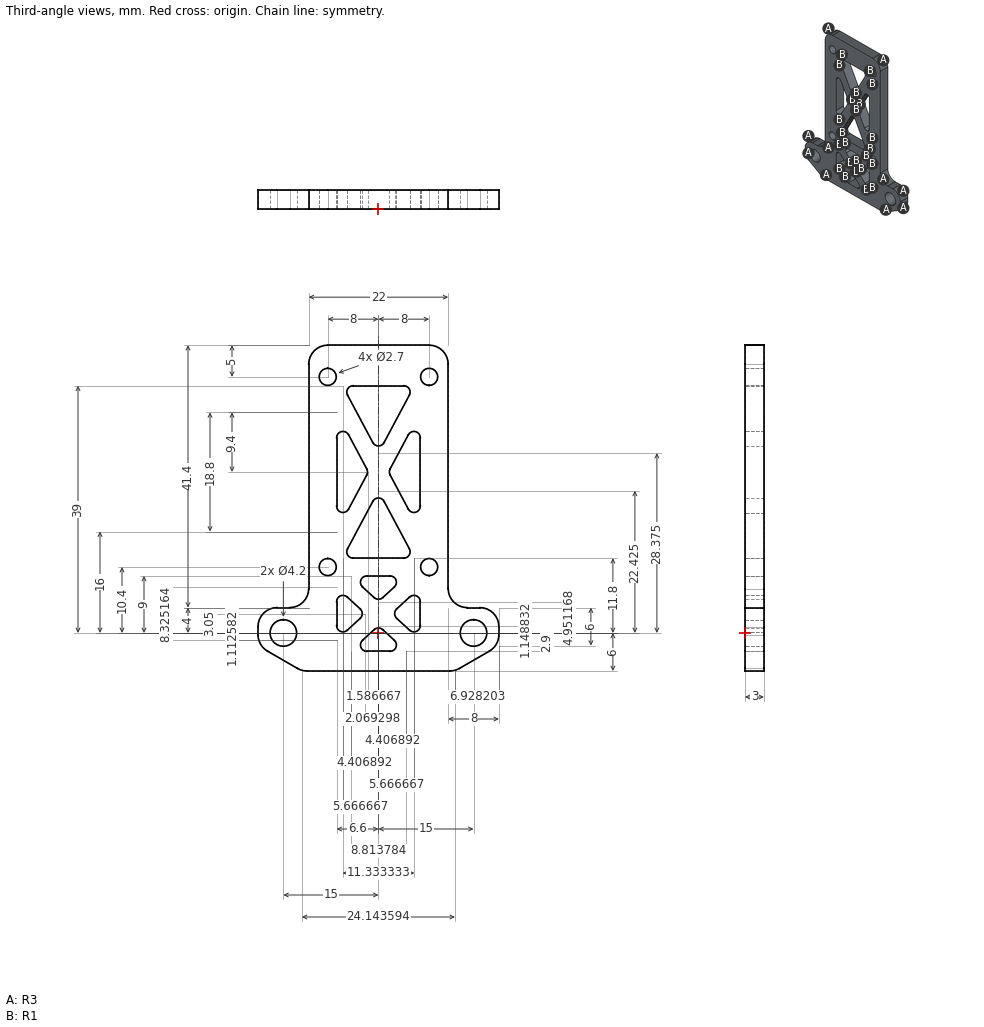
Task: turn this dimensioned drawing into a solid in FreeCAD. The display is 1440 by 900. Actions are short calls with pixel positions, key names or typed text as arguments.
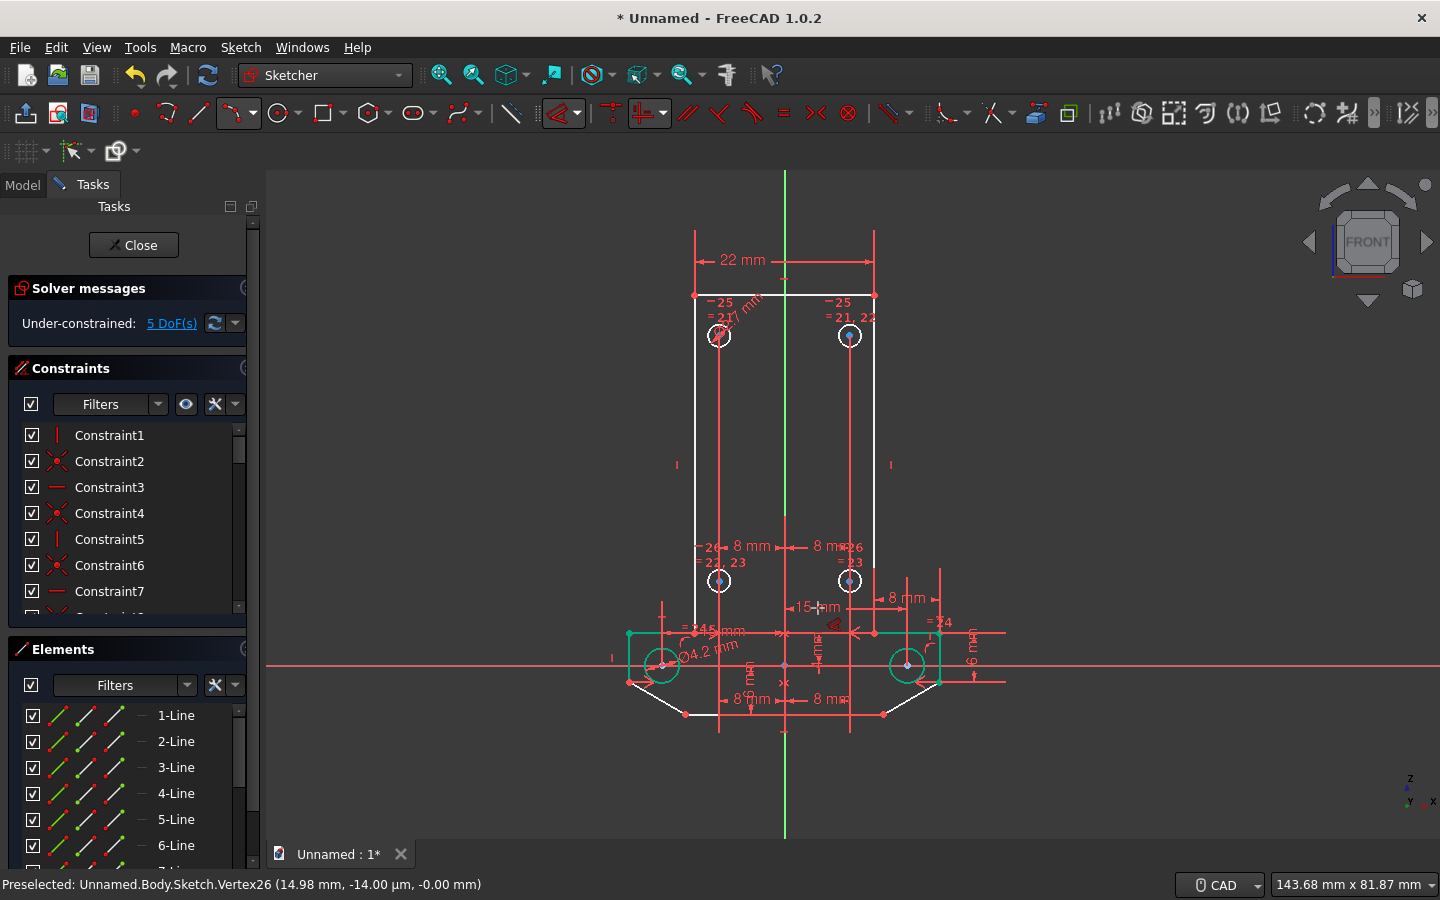
click(695, 295)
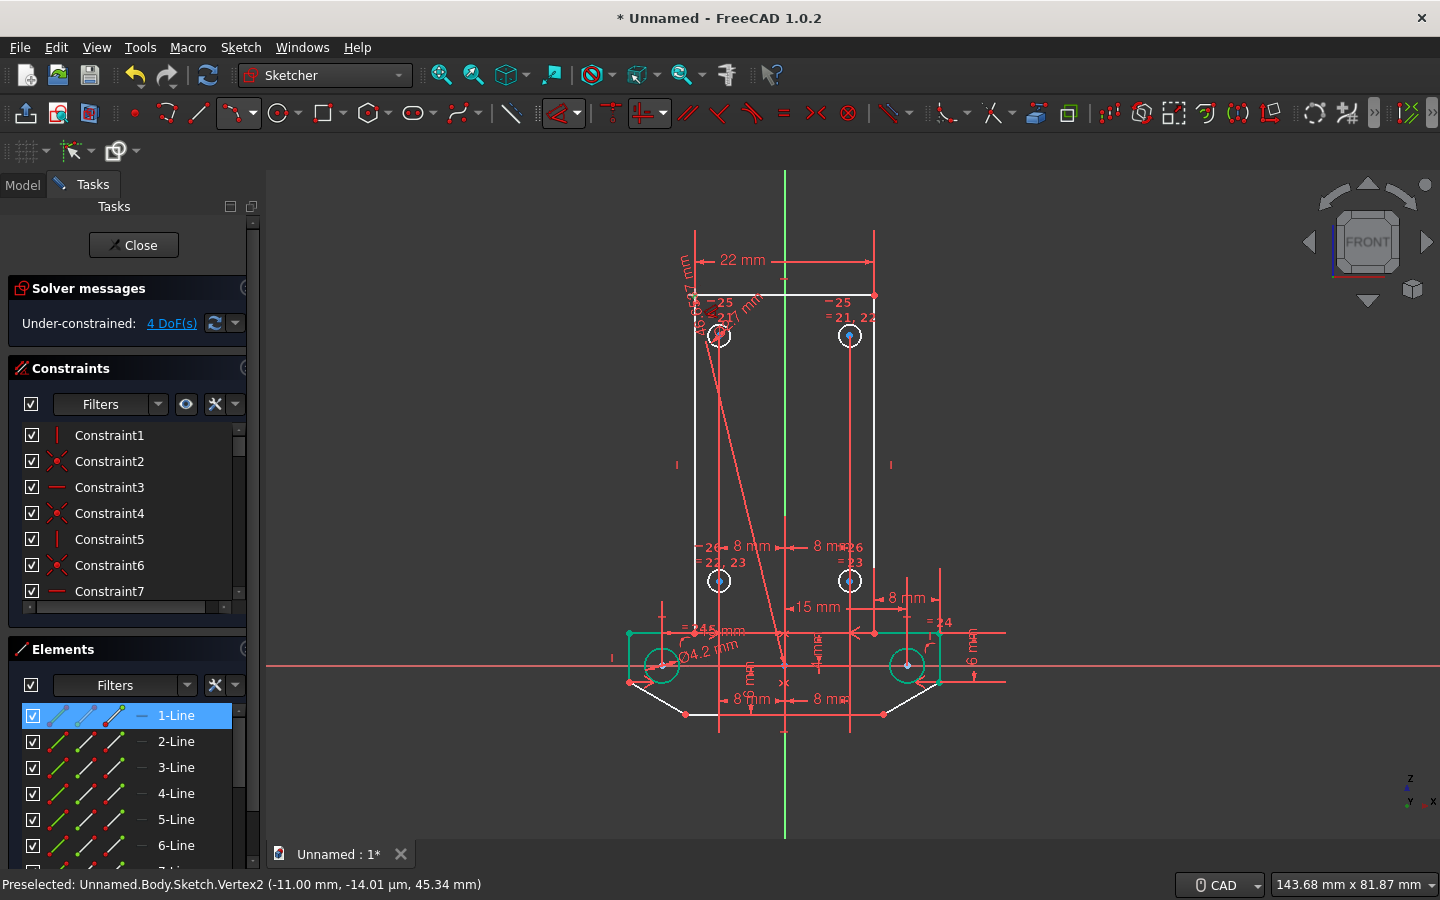
click(719, 336)
click(661, 316)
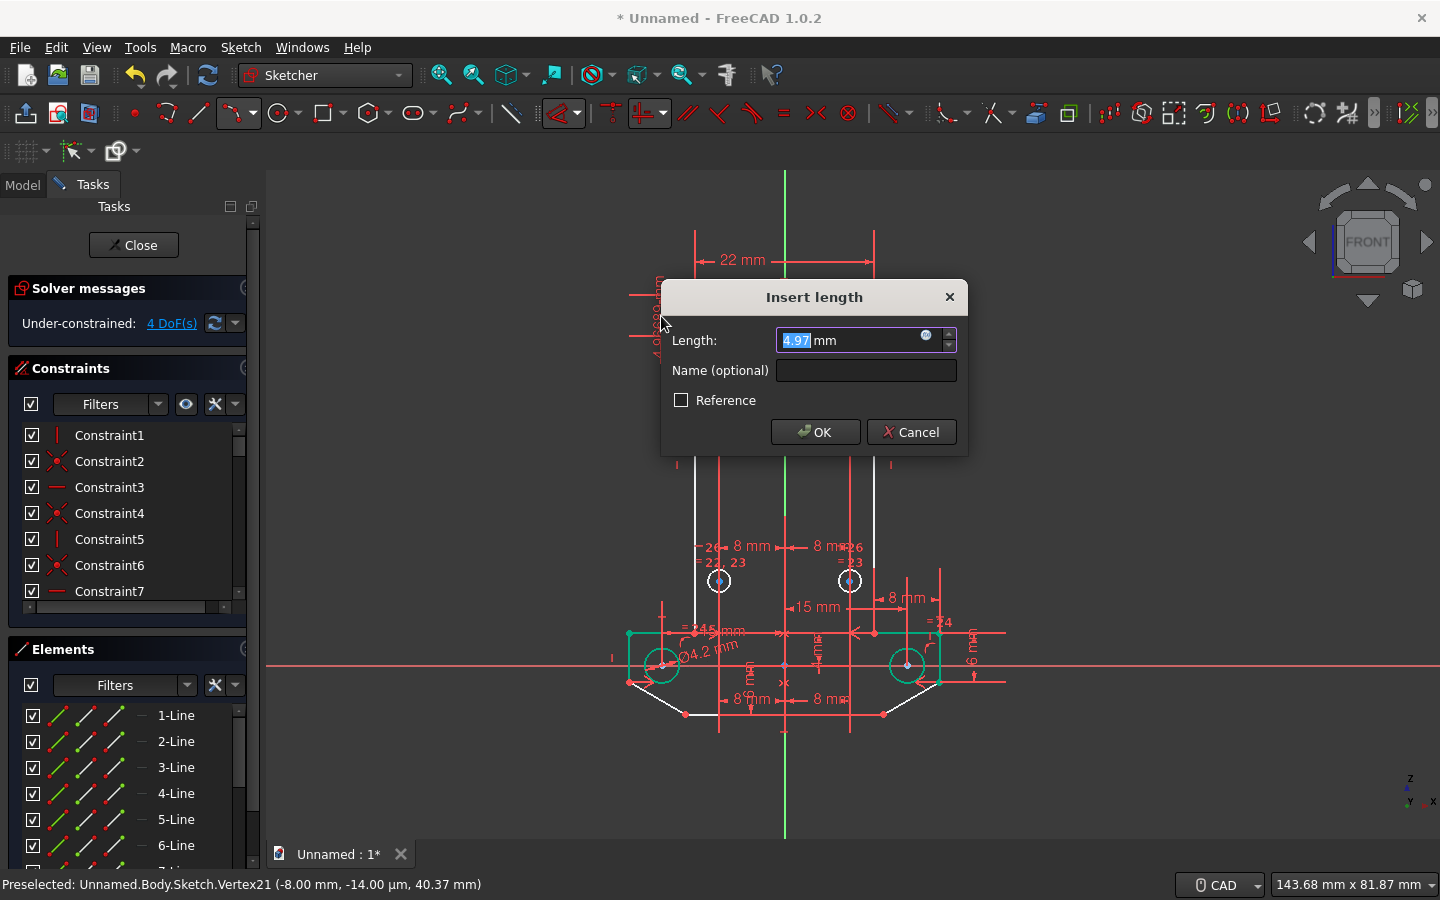
text(5)
key(Return)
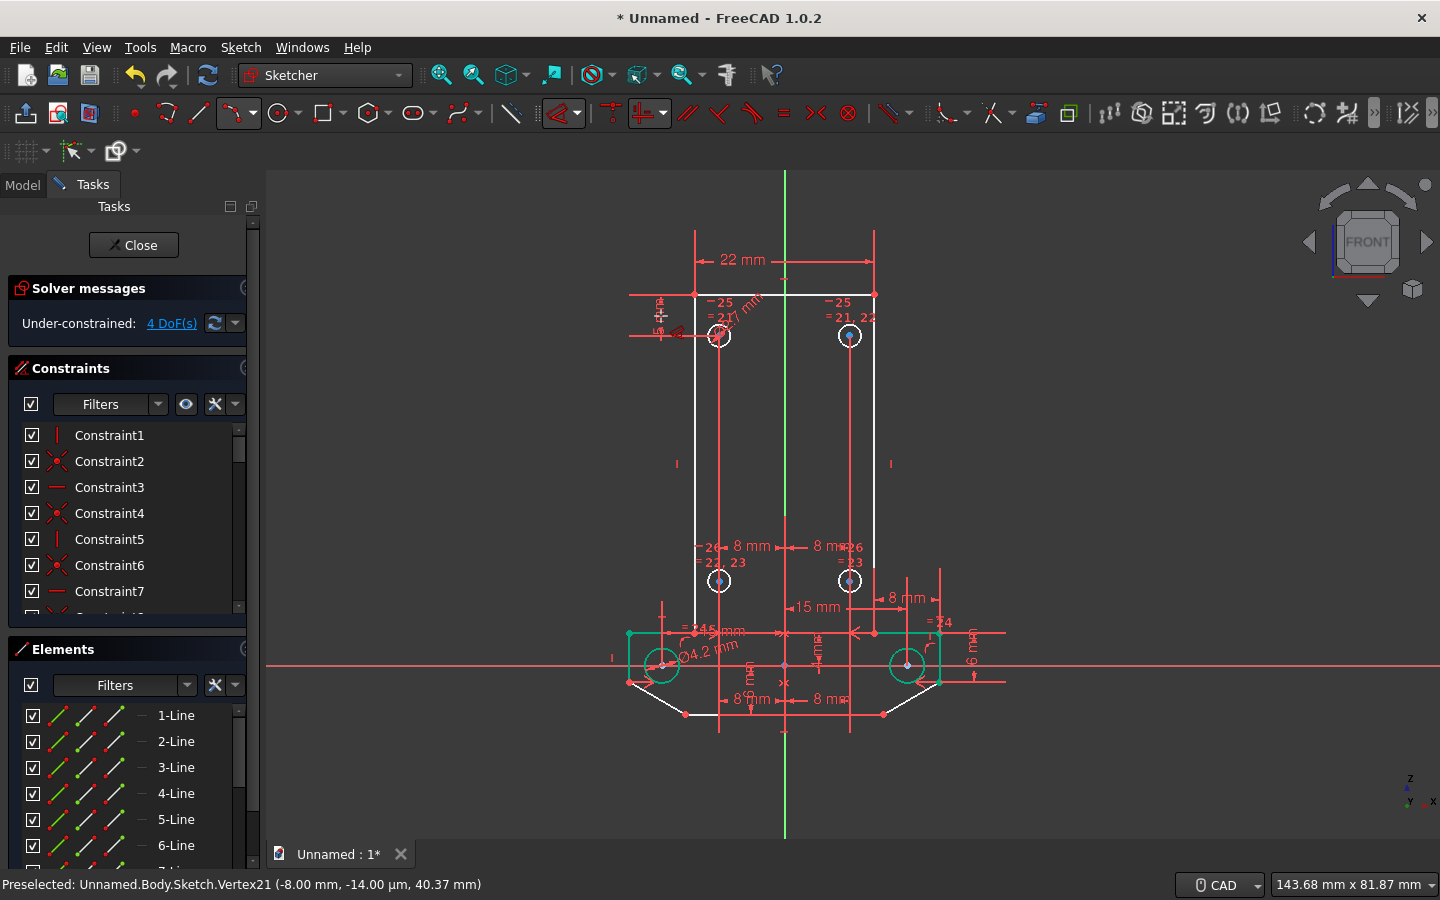
click(695, 532)
click(661, 464)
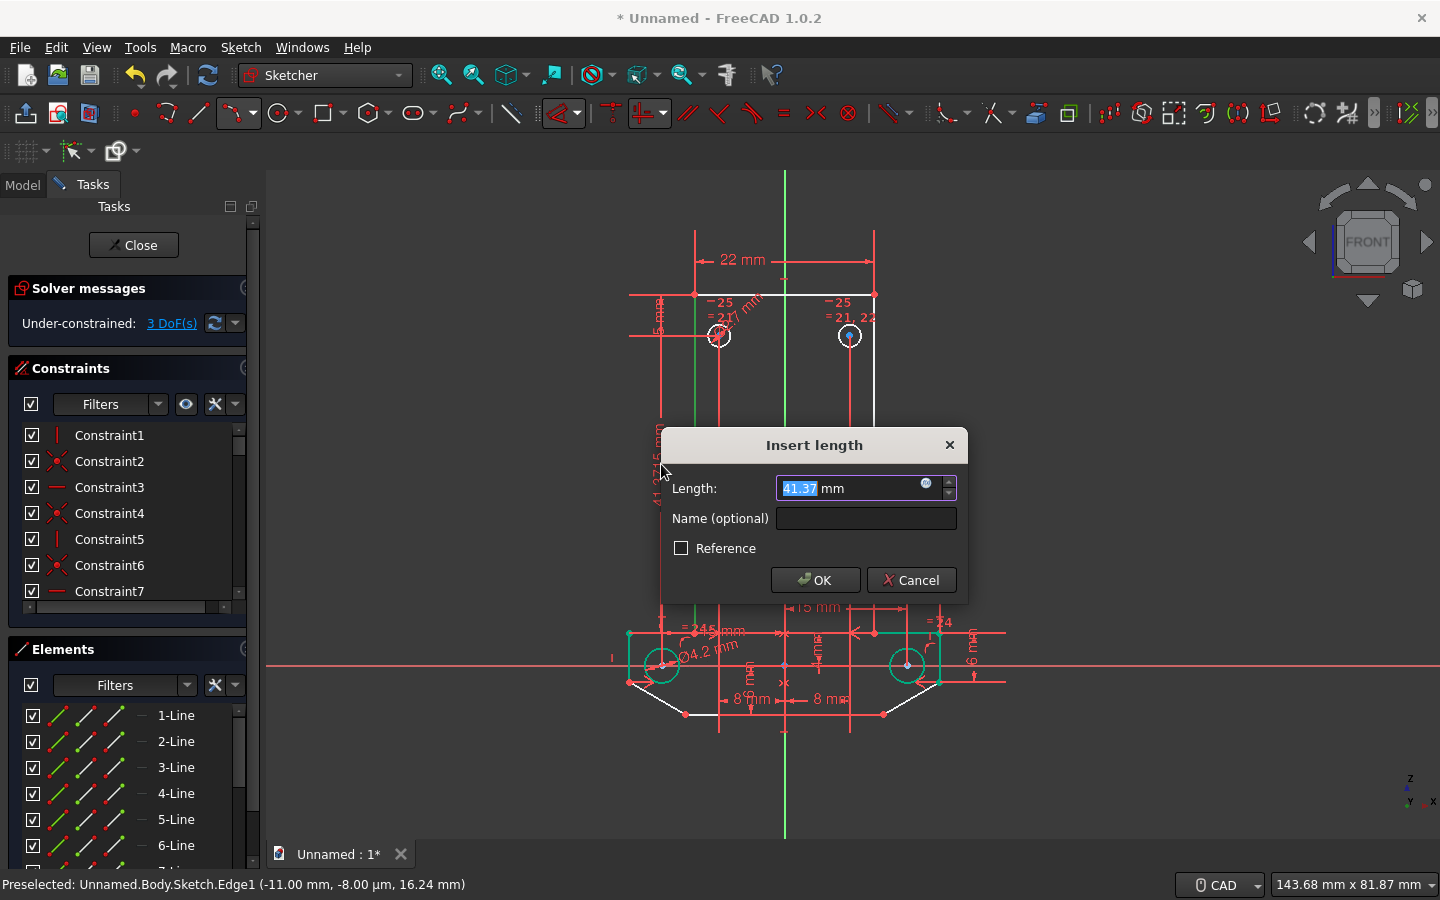
text(41.4)
key(Return)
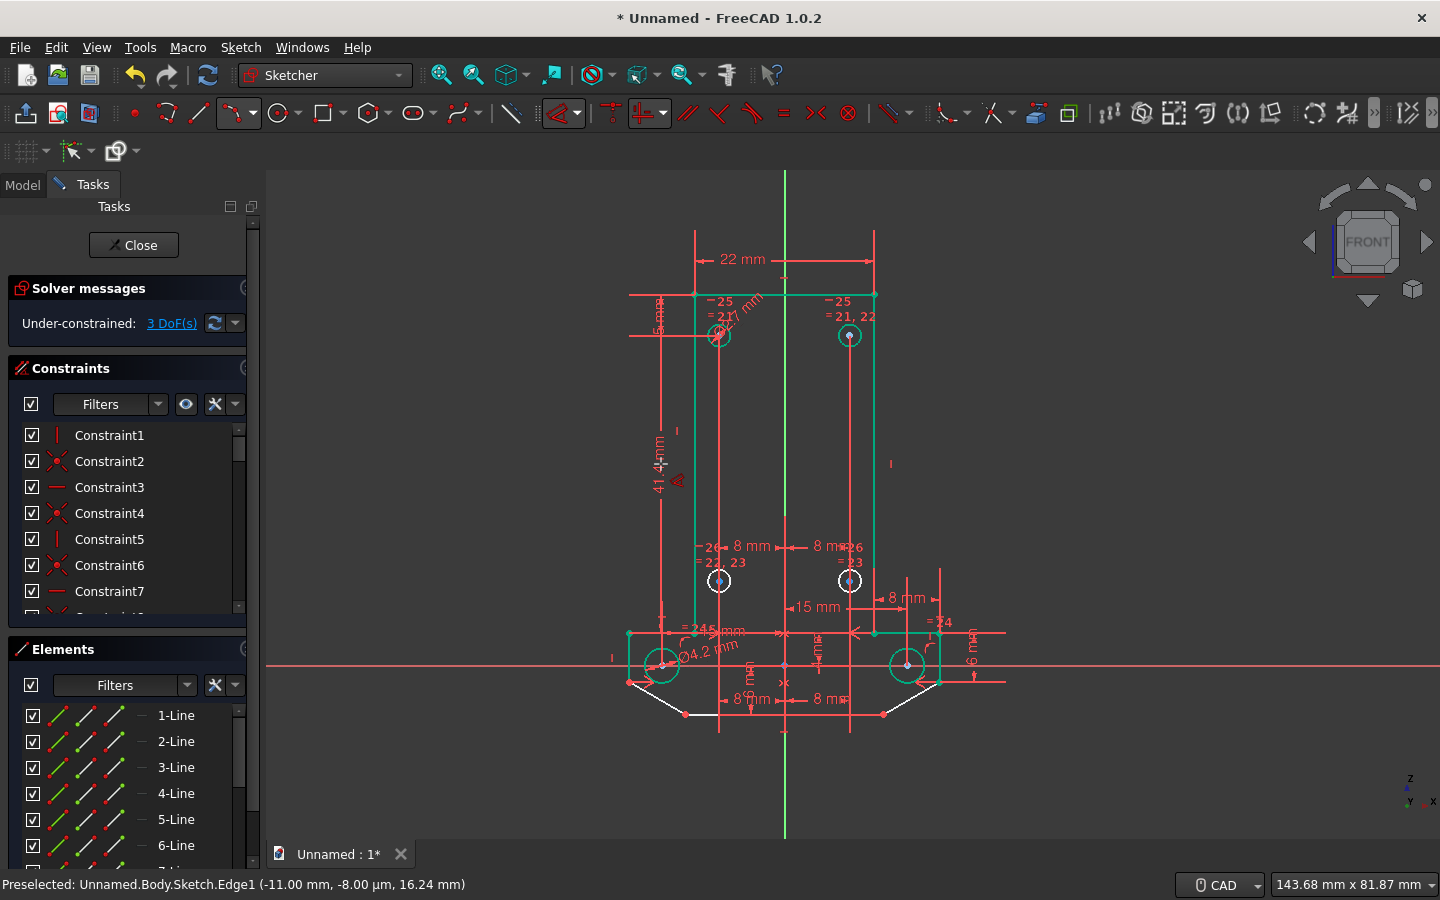
click(719, 581)
click(661, 604)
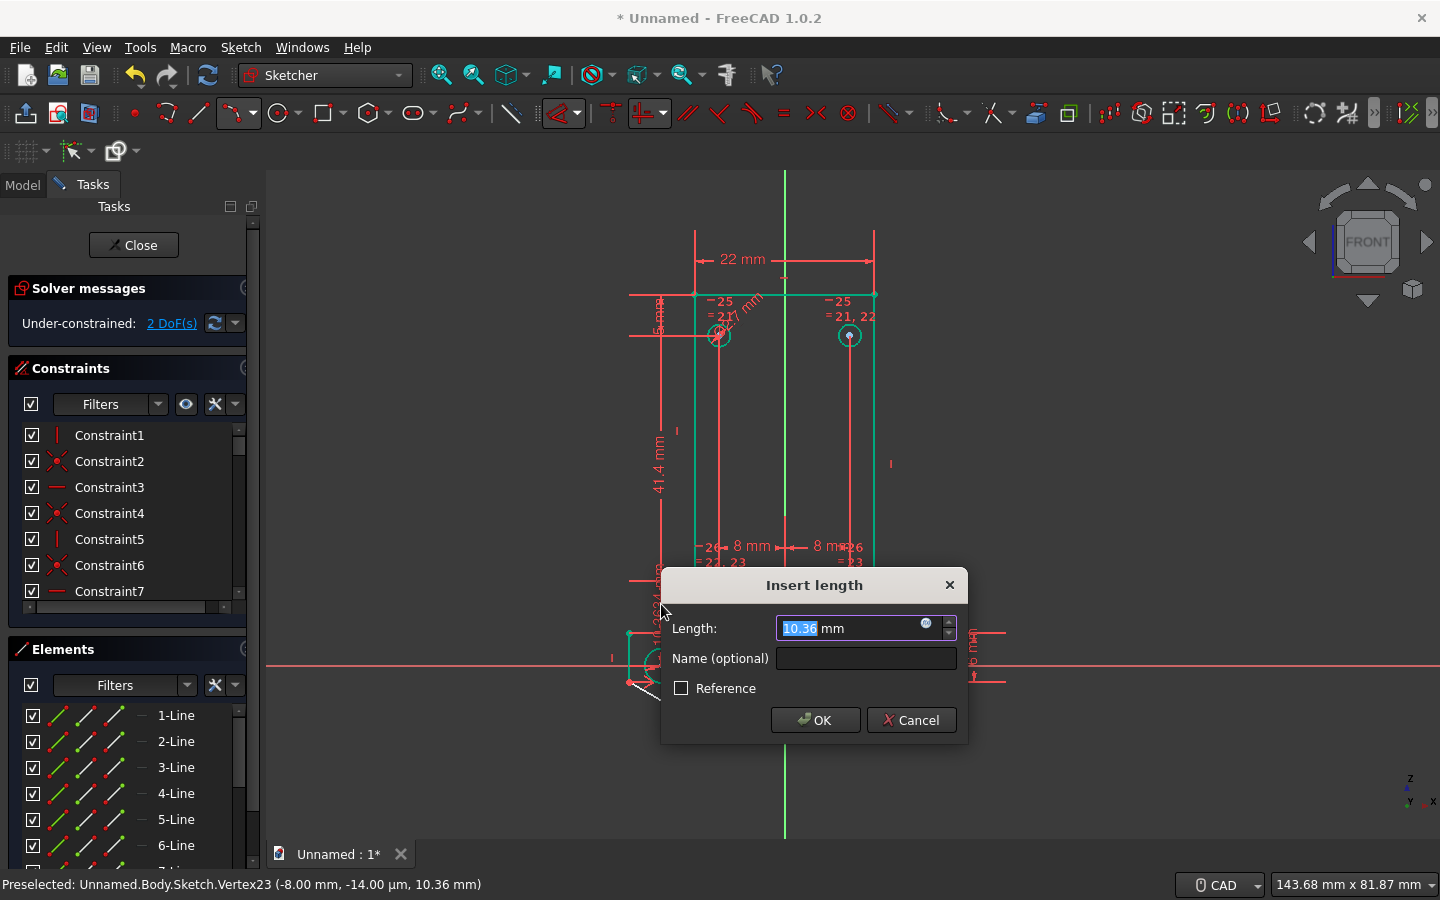
text(10.4)
key(Return)